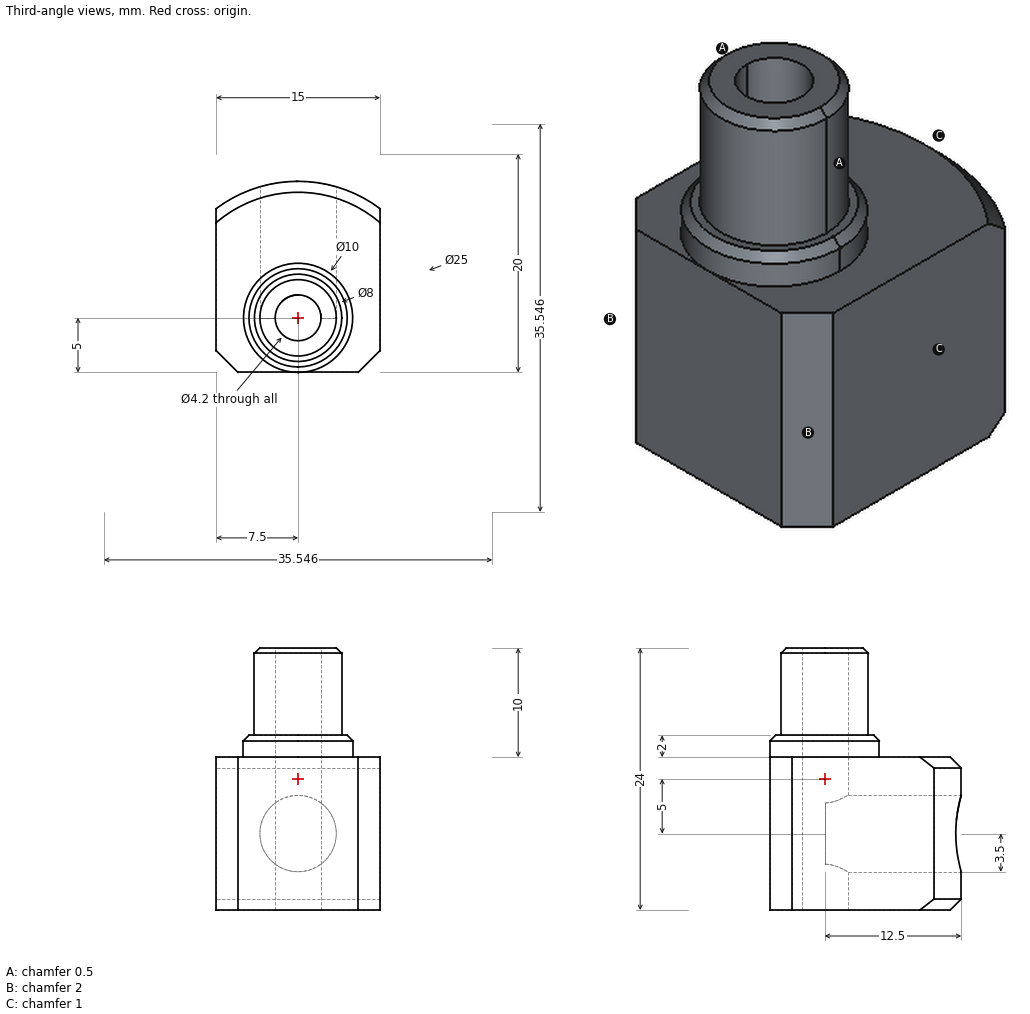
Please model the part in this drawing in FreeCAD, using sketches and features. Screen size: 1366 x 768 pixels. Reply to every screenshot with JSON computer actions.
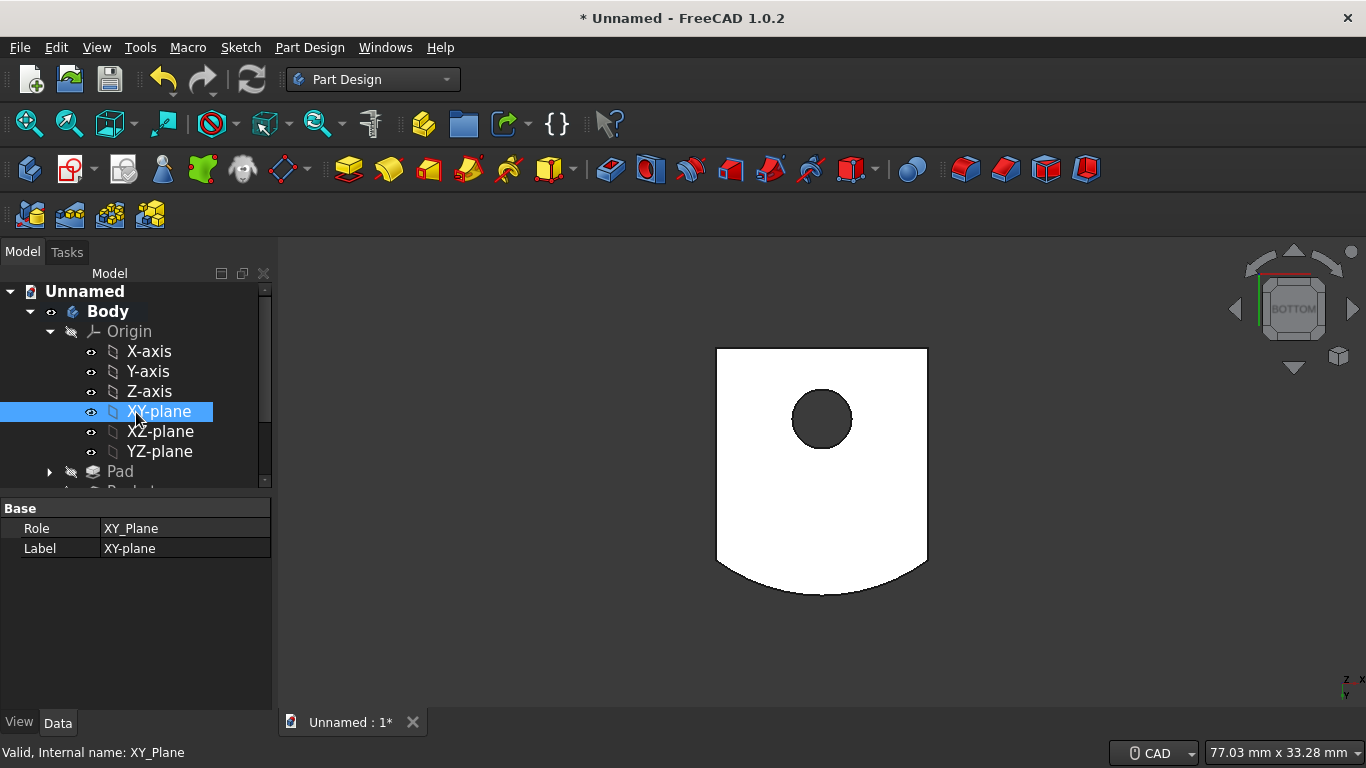
{"action": "left_click", "coordinate": [284, 170]}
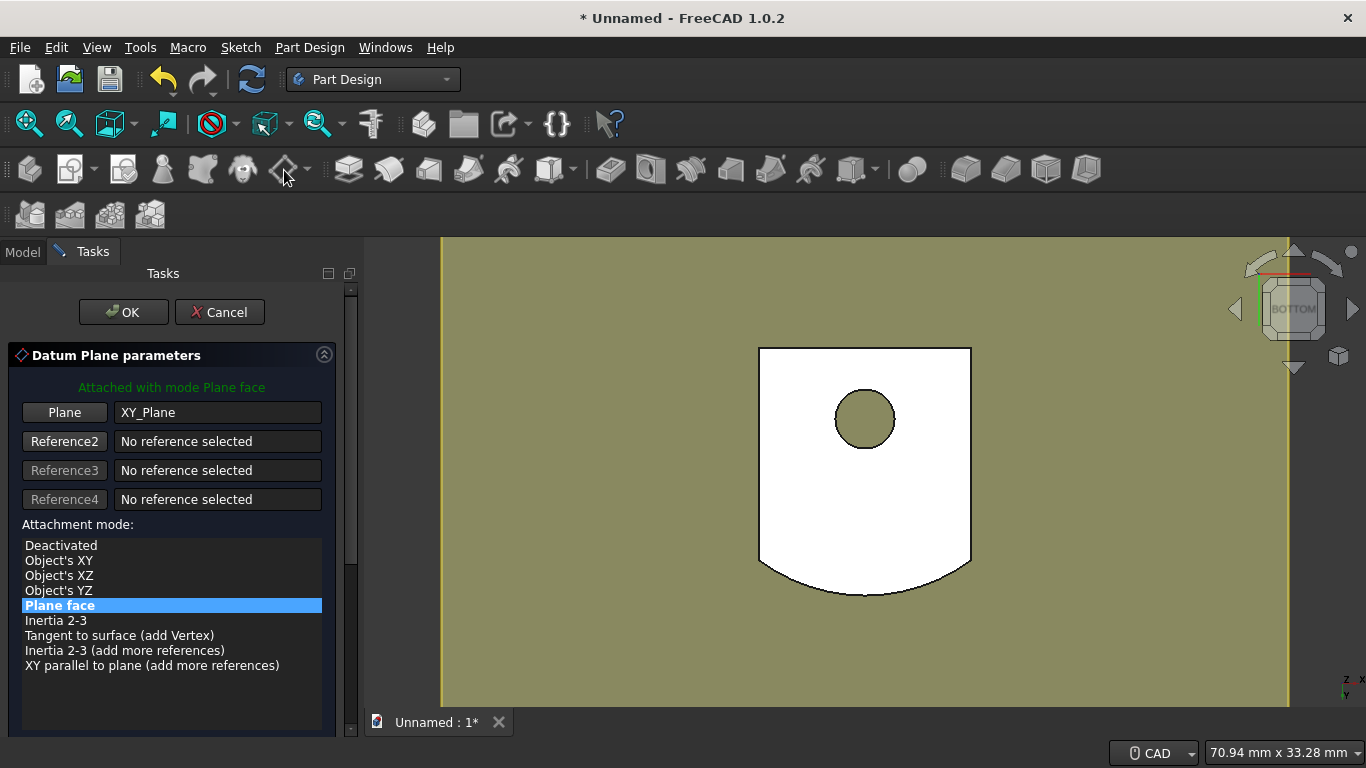
{"action": "scroll", "coordinate": [351, 510], "scroll_direction": "down", "scroll_amount": 3}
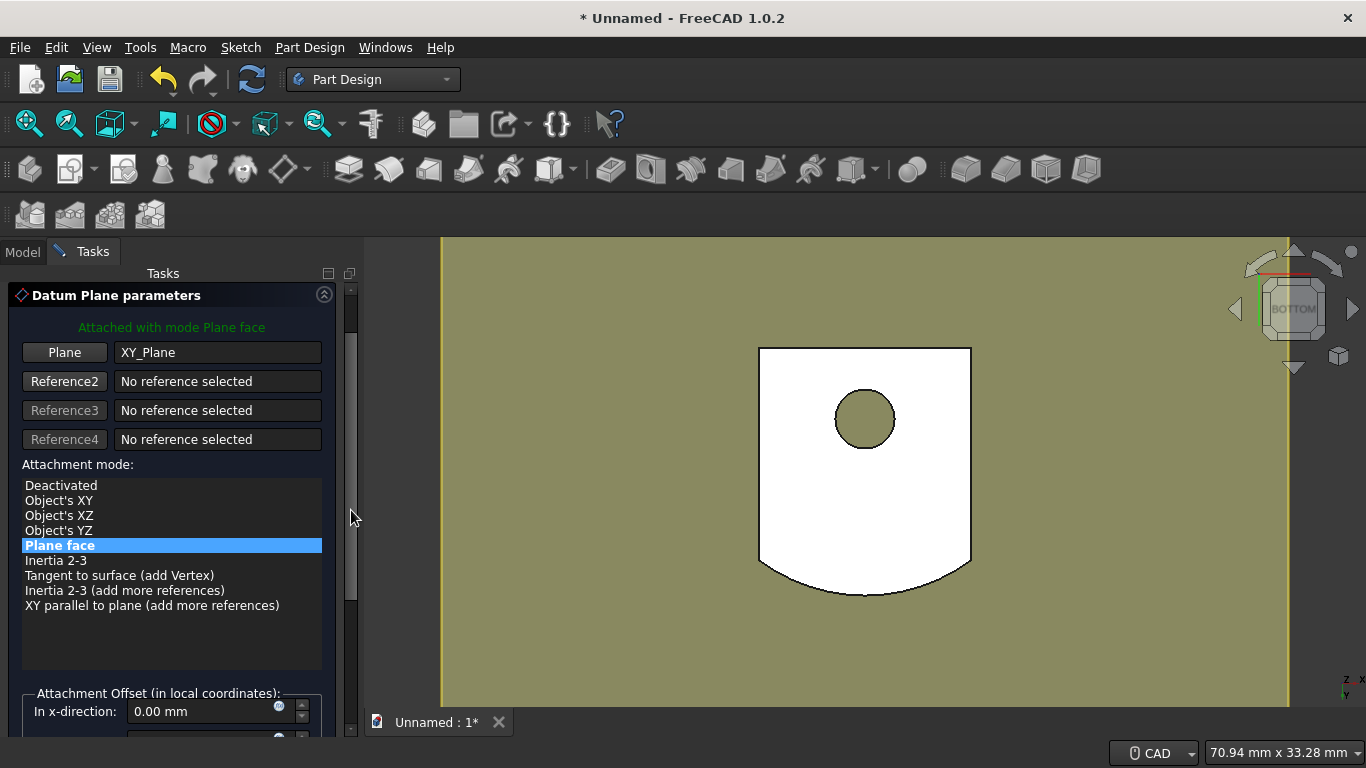
{"action": "triple_click", "coordinate": [210, 655]}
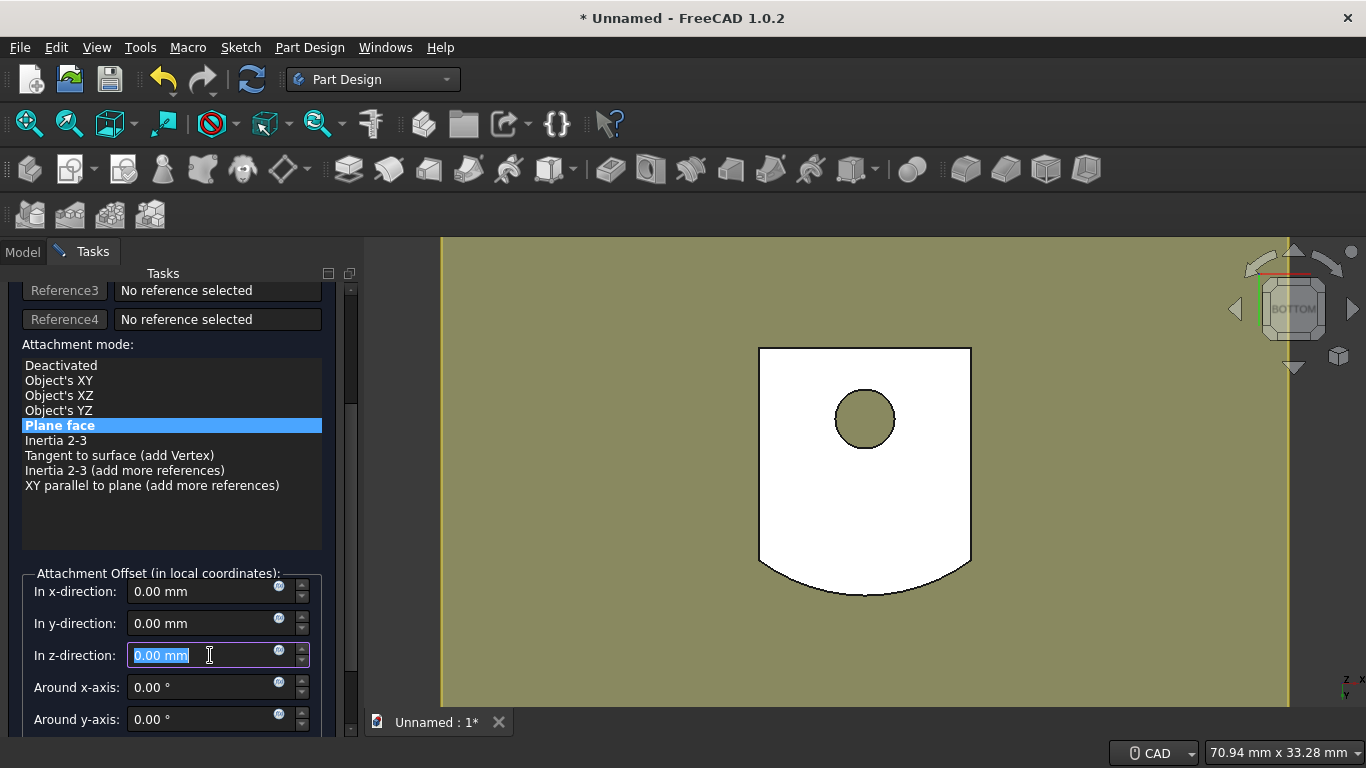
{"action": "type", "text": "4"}
{"action": "key", "text": "Tab"}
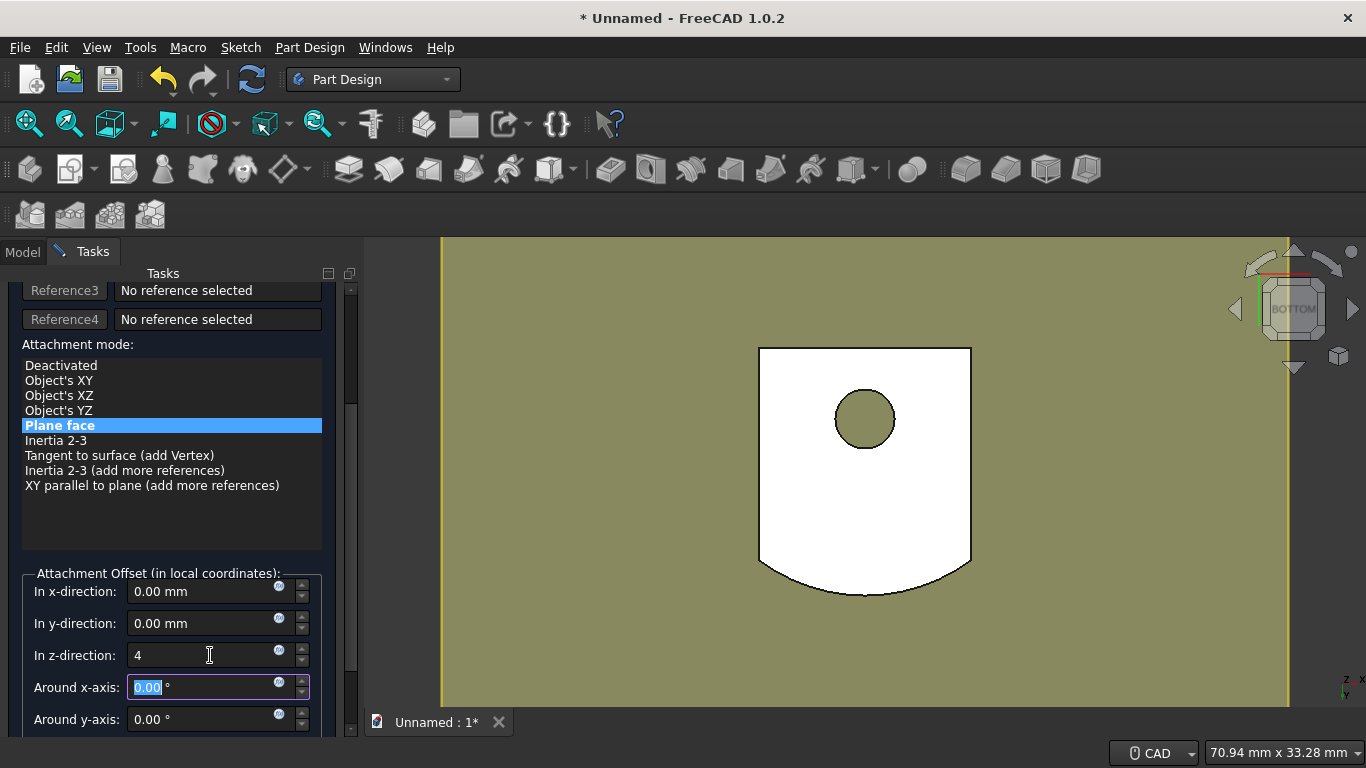
{"action": "scroll", "coordinate": [351, 510], "scroll_direction": "up", "scroll_amount": 4}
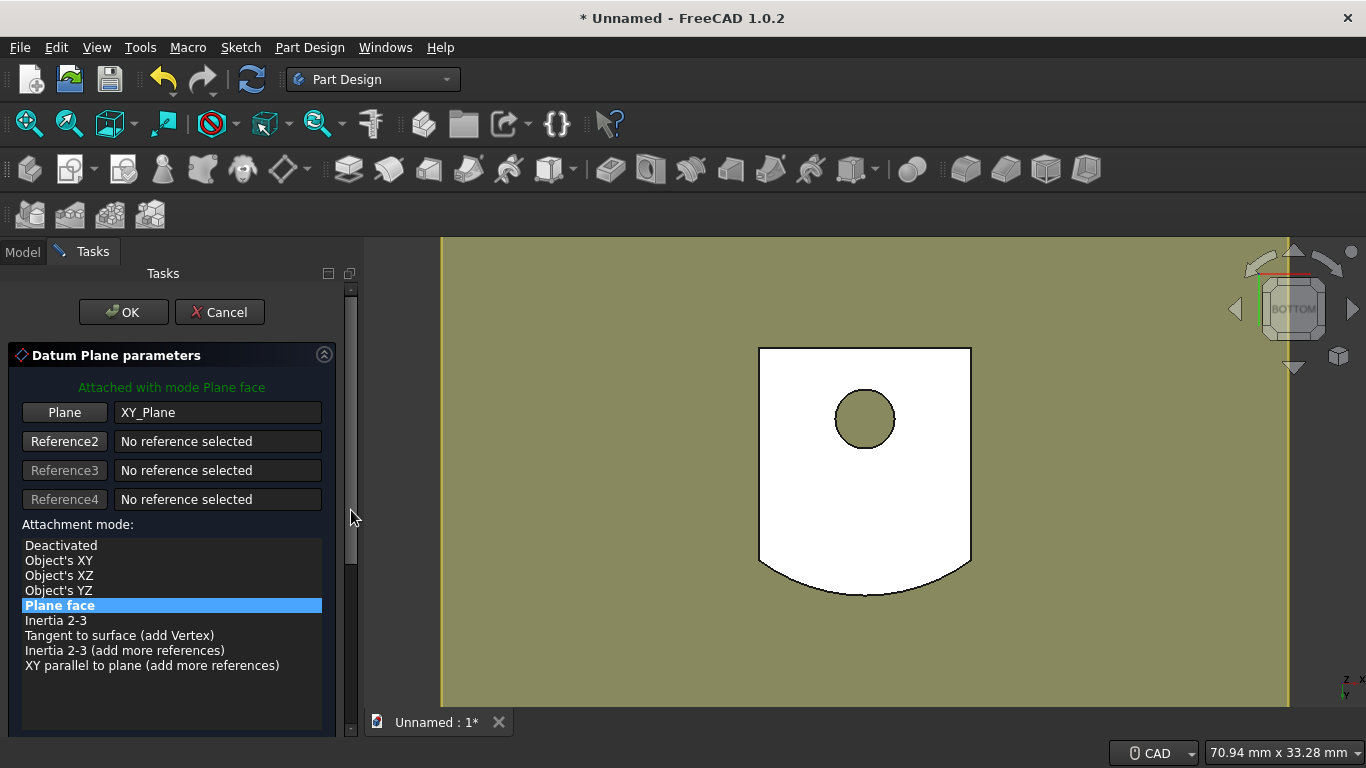
{"action": "left_click", "coordinate": [124, 312]}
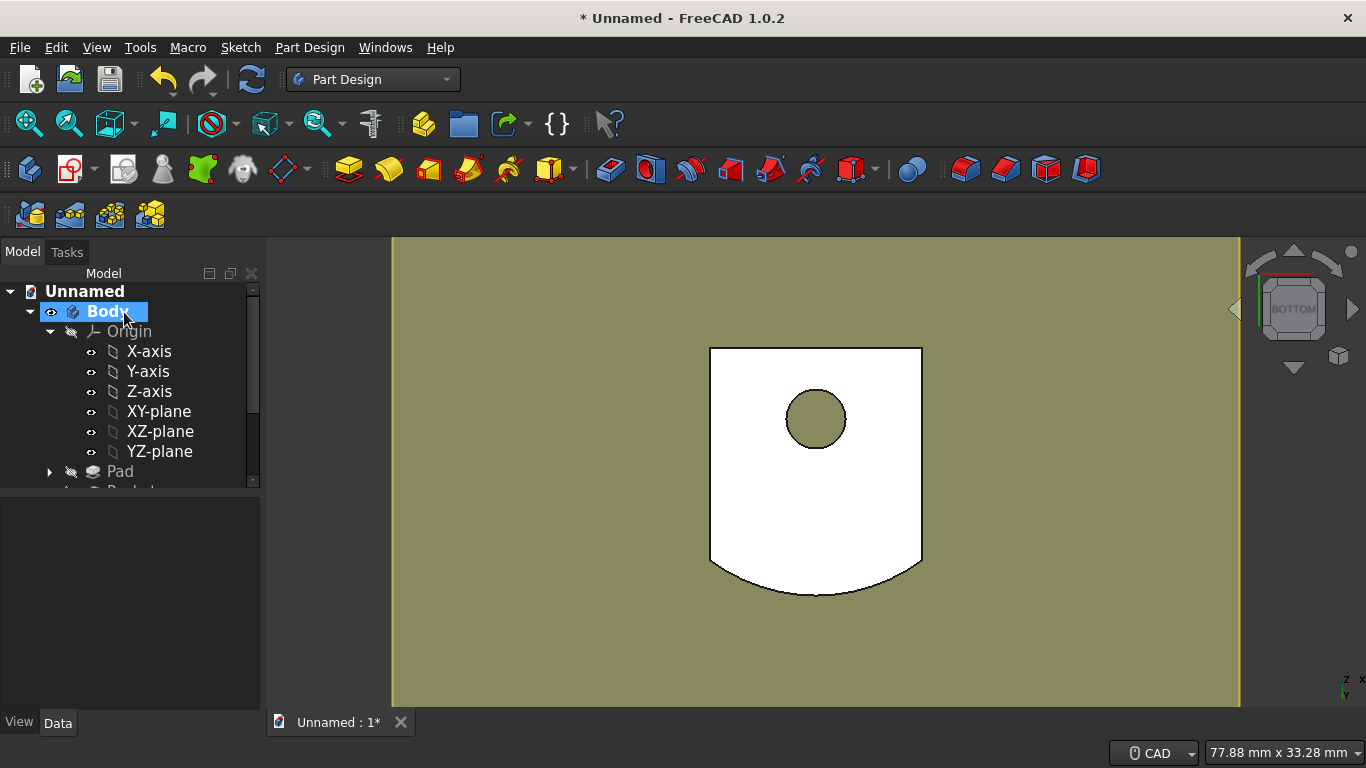
{"action": "scroll", "coordinate": [100, 387], "scroll_direction": "down", "scroll_amount": 3}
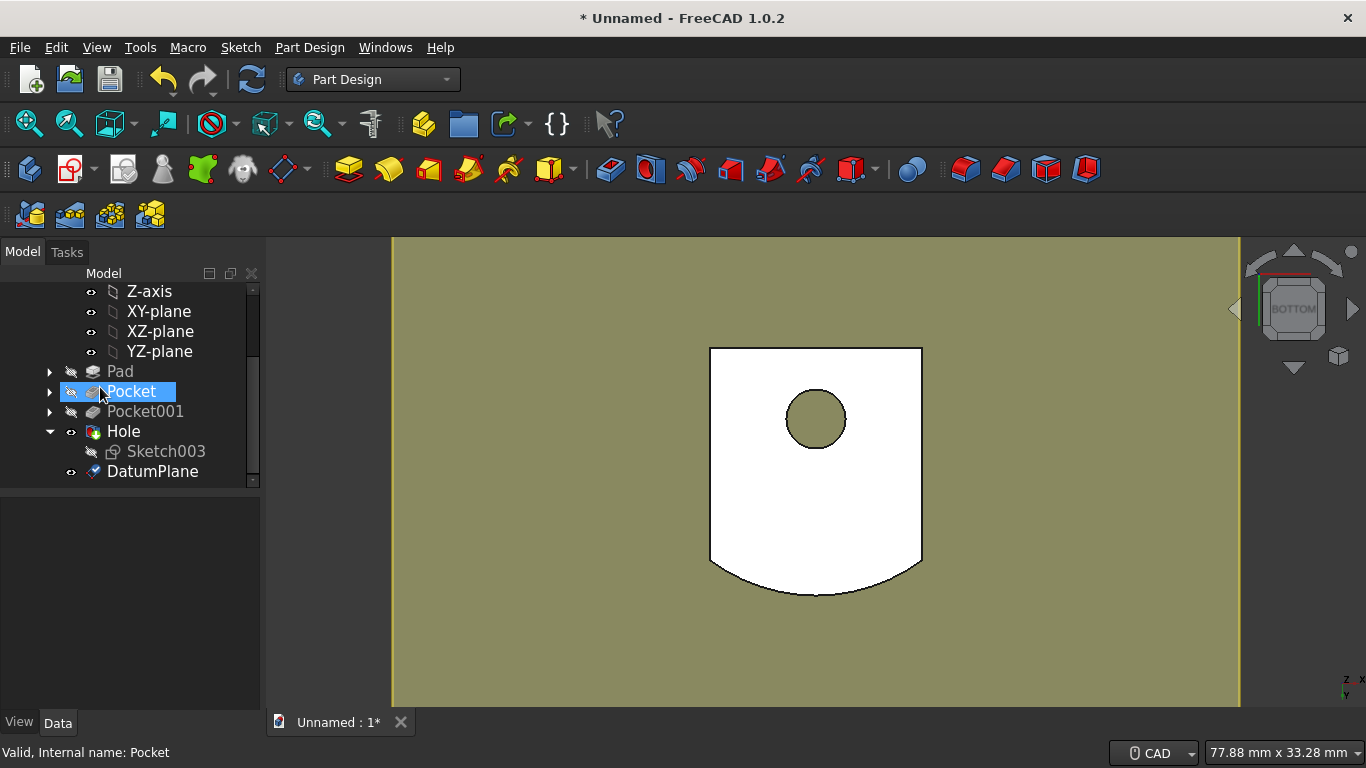
{"action": "left_click", "coordinate": [116, 472]}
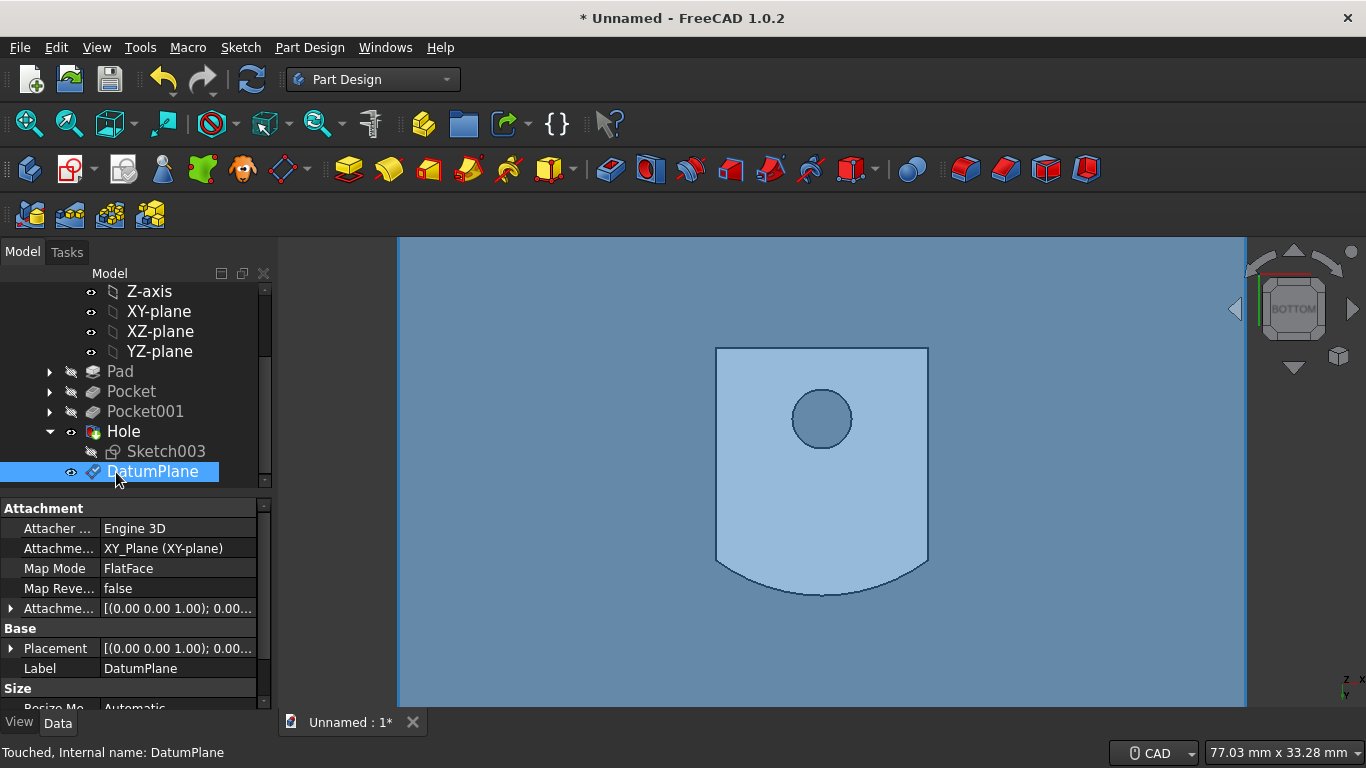
{"action": "left_click", "coordinate": [70, 170]}